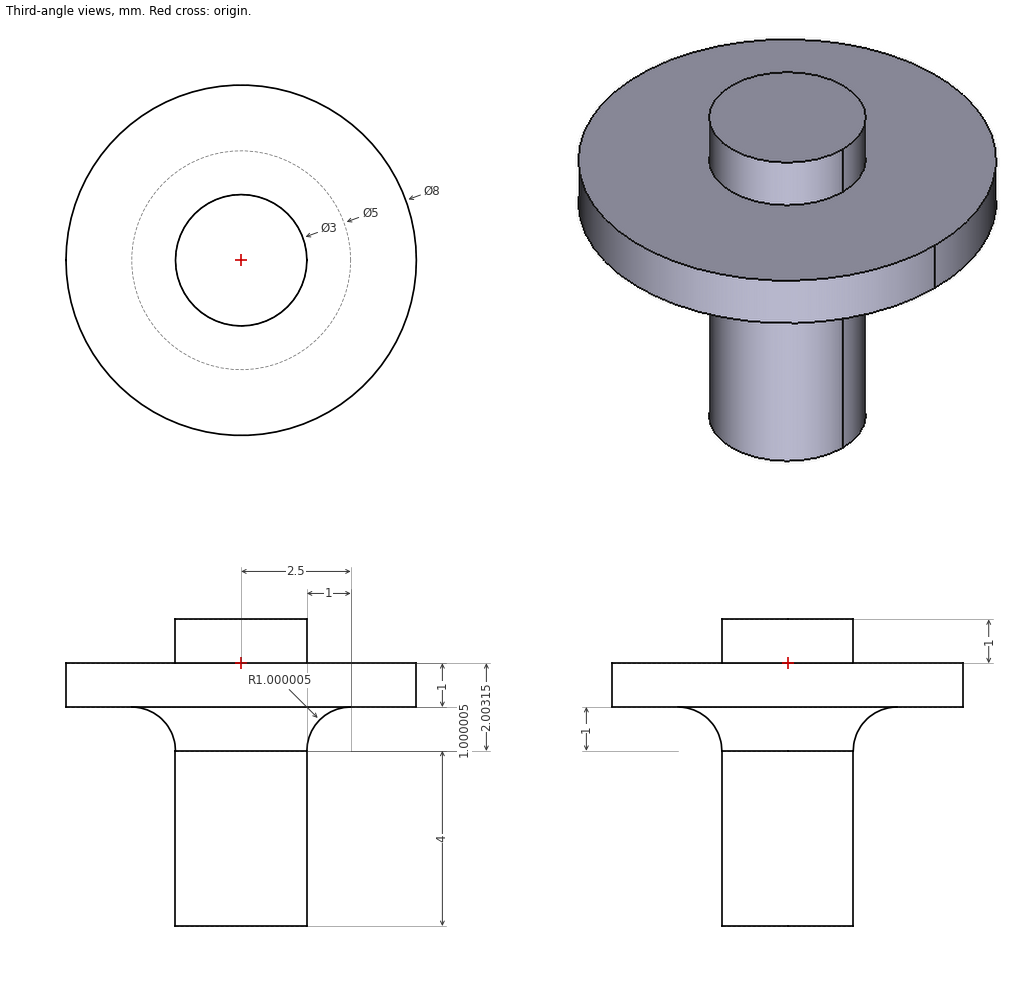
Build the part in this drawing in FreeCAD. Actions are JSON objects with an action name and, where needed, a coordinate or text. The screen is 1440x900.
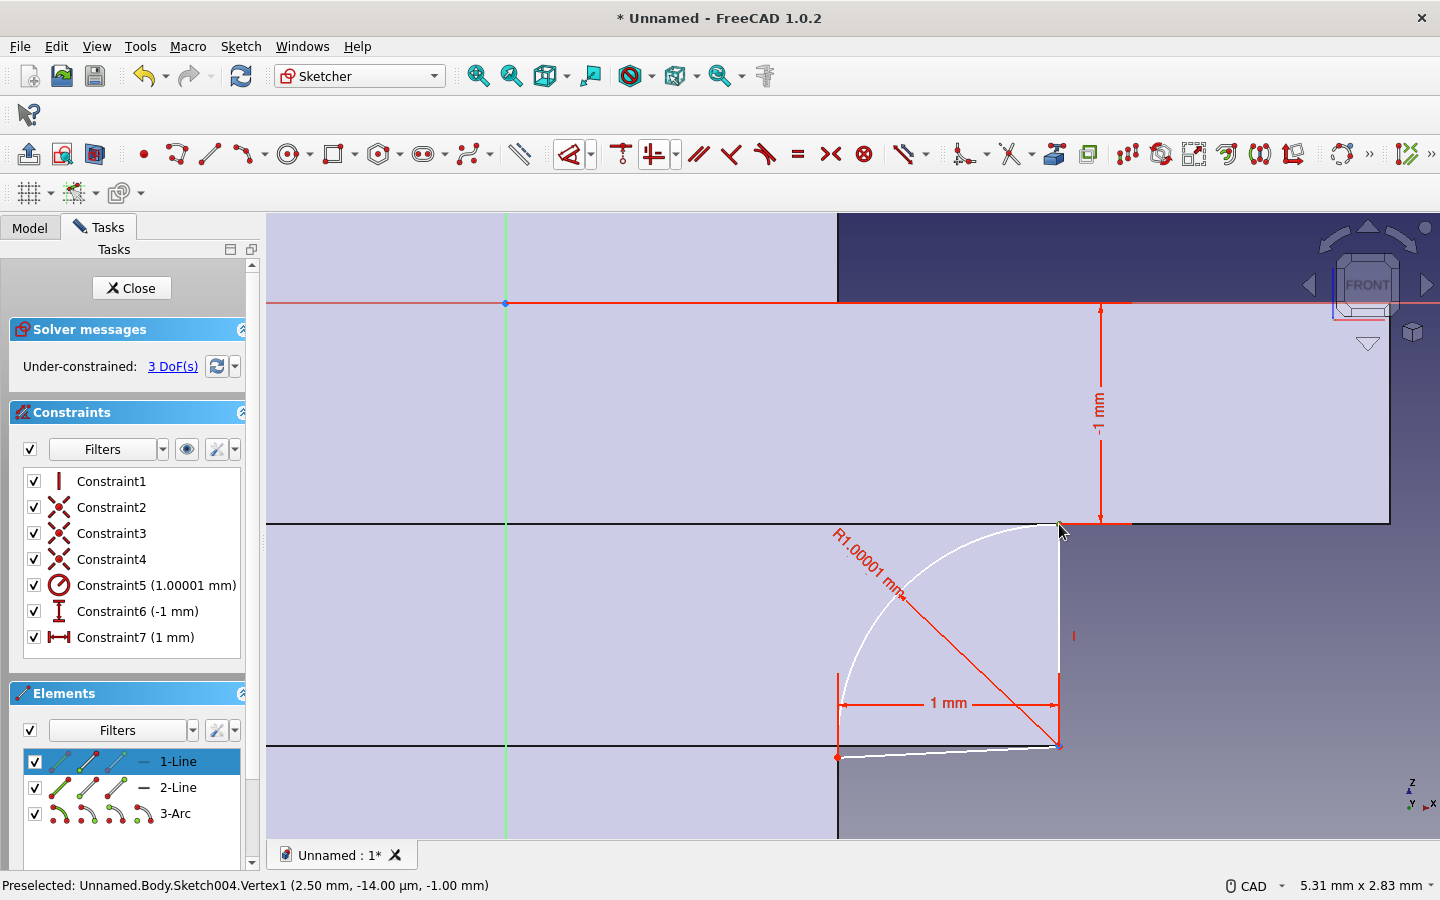
{"action": "key", "text": "l"}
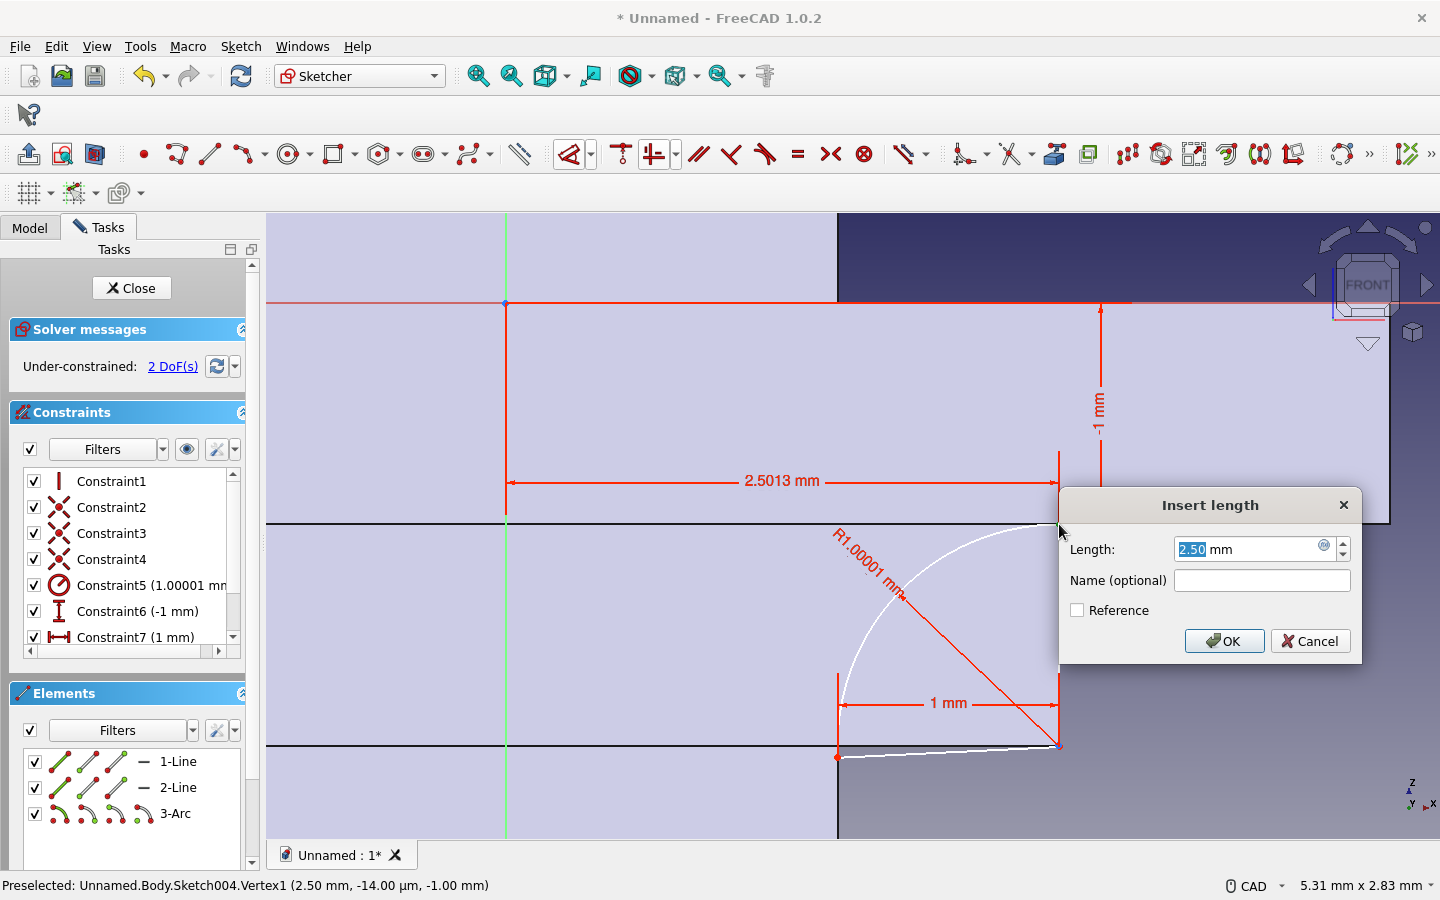
{"action": "type", "text": "2.5"}
{"action": "key", "text": "Return"}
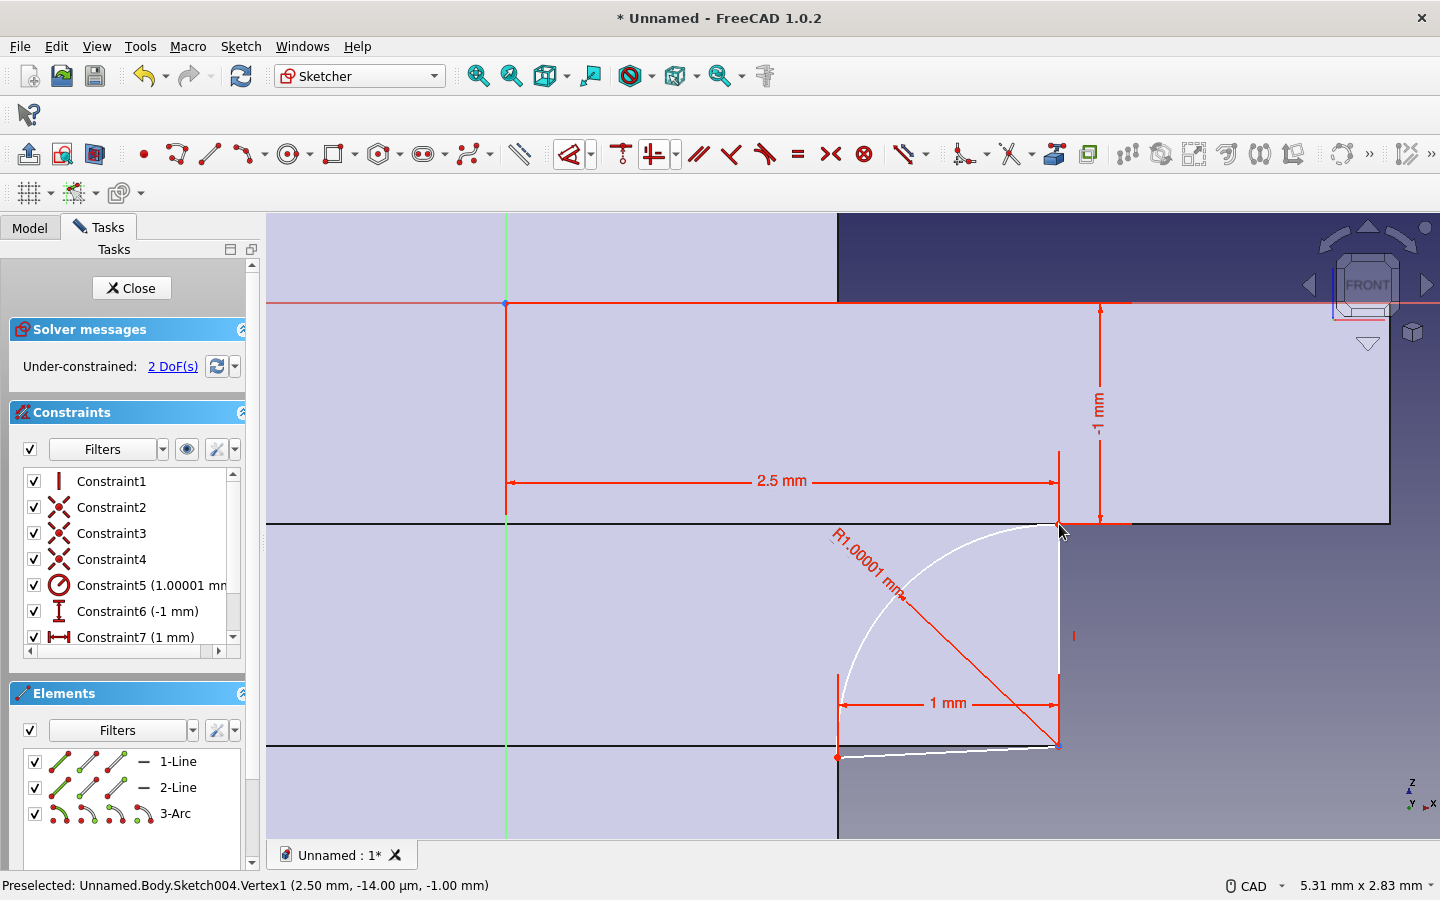
{"action": "left_click", "coordinate": [1059, 591]}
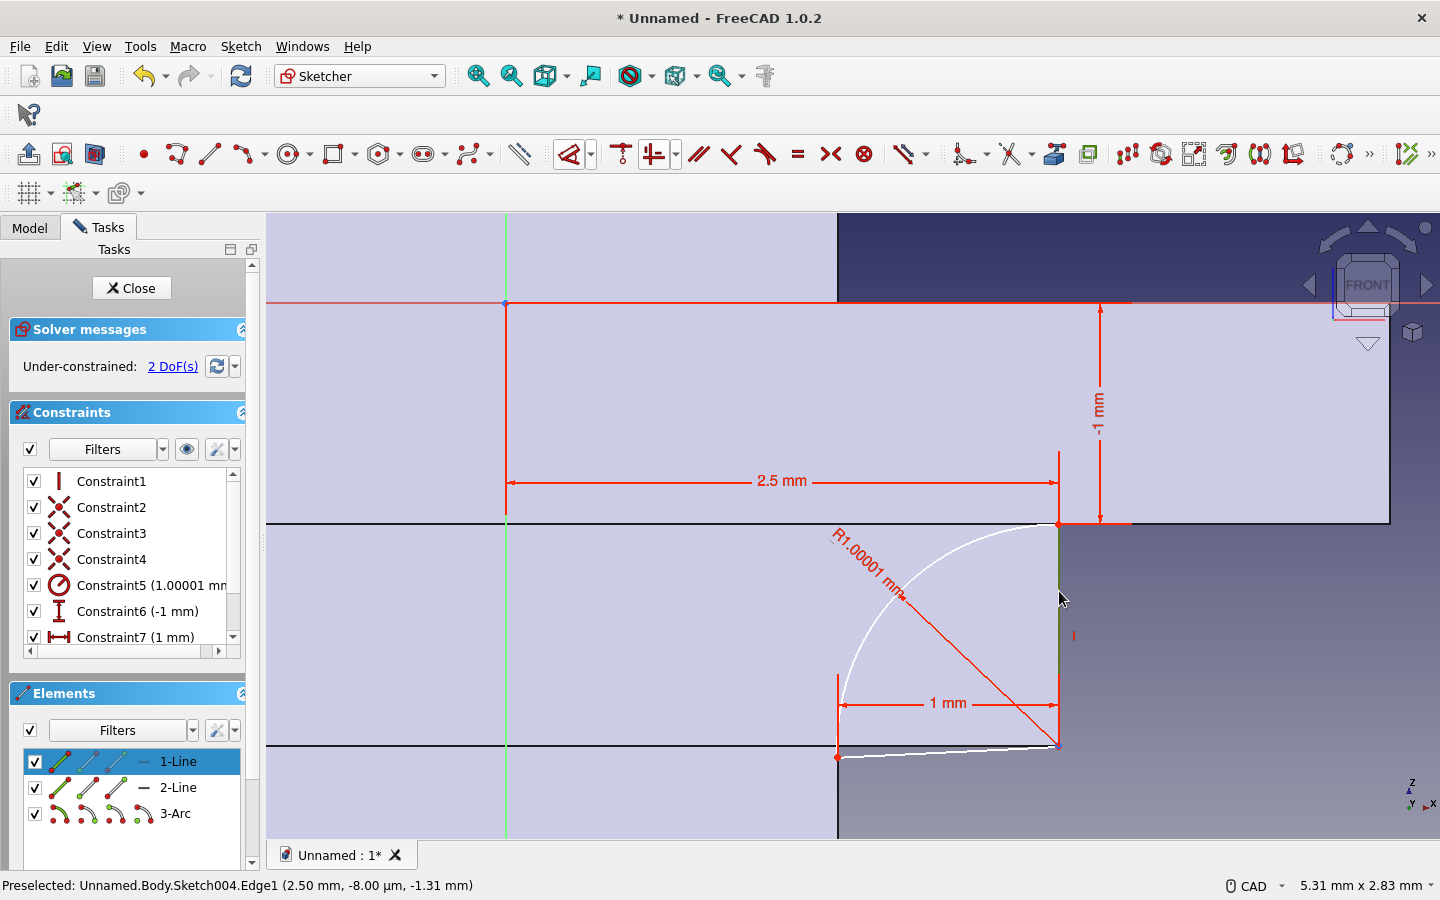
{"action": "left_click", "coordinate": [590, 154]}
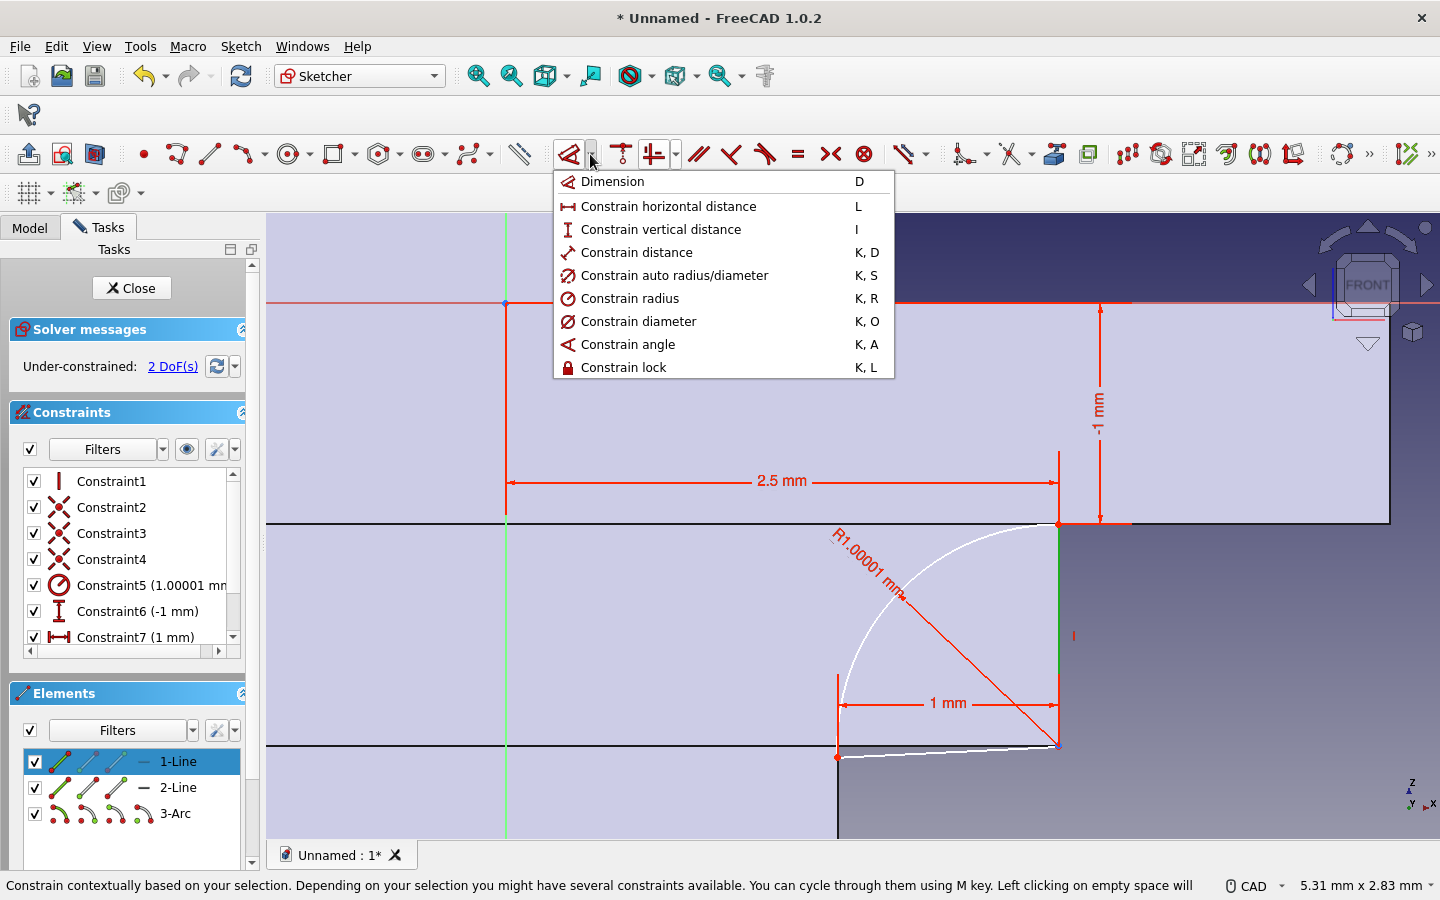
{"action": "left_click", "coordinate": [724, 230]}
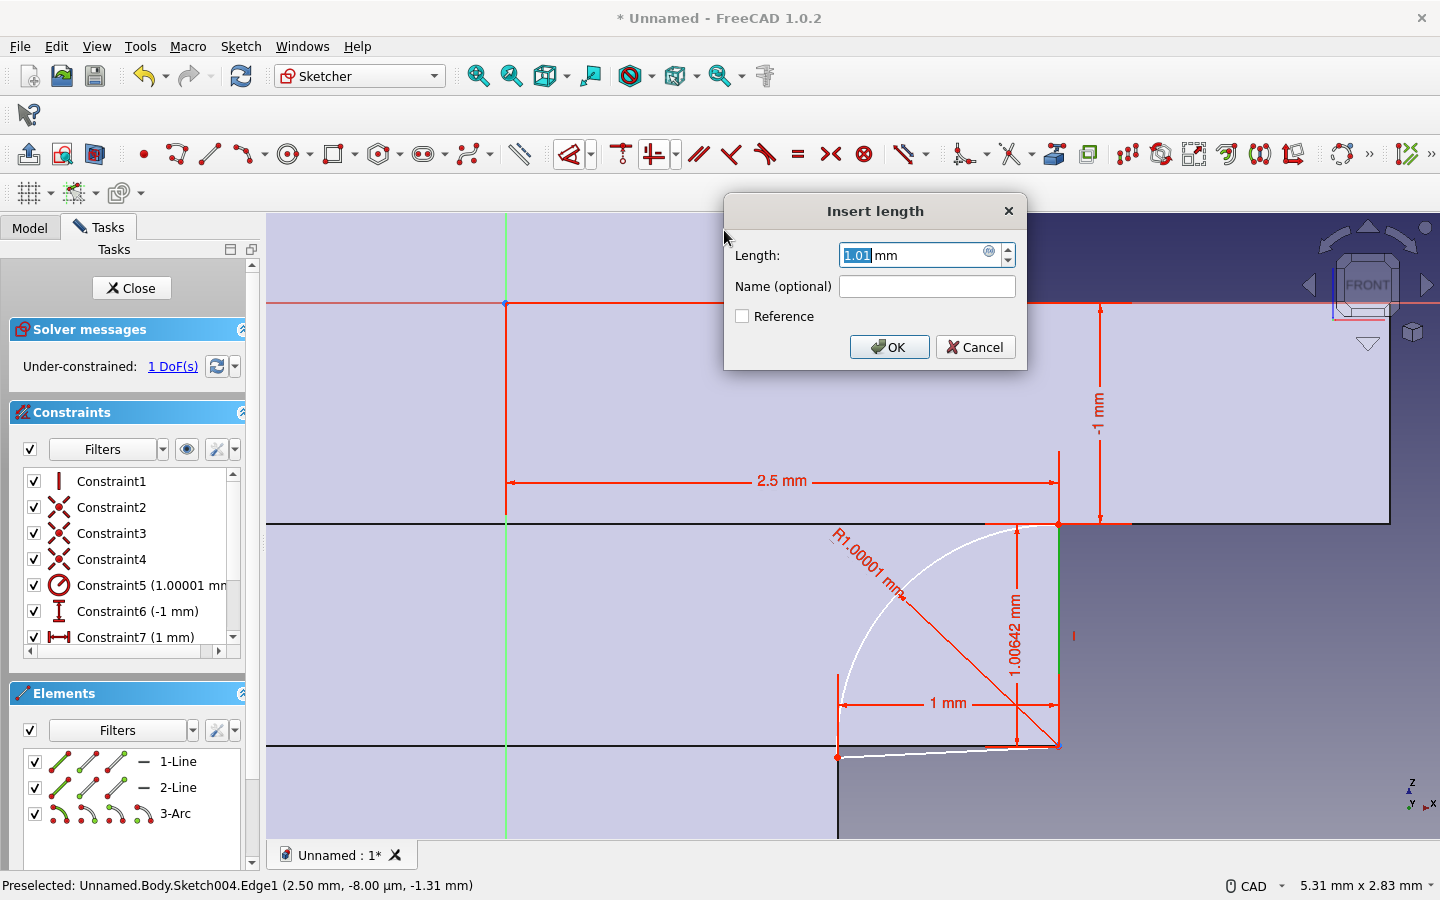
{"action": "type", "text": "1.000005"}
{"action": "key", "text": "Return"}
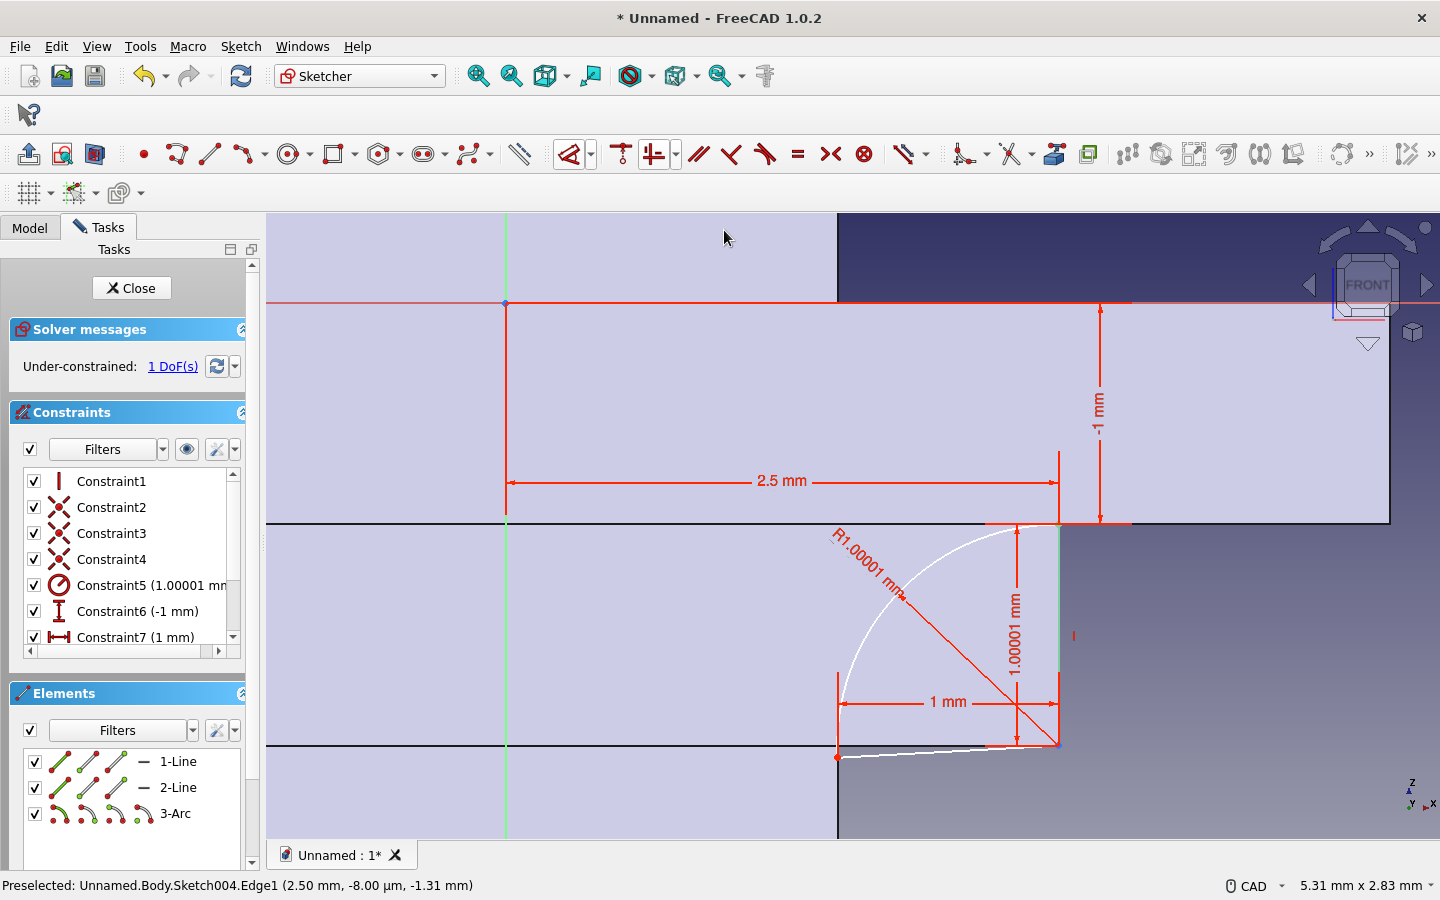
{"action": "left_click", "coordinate": [838, 758]}